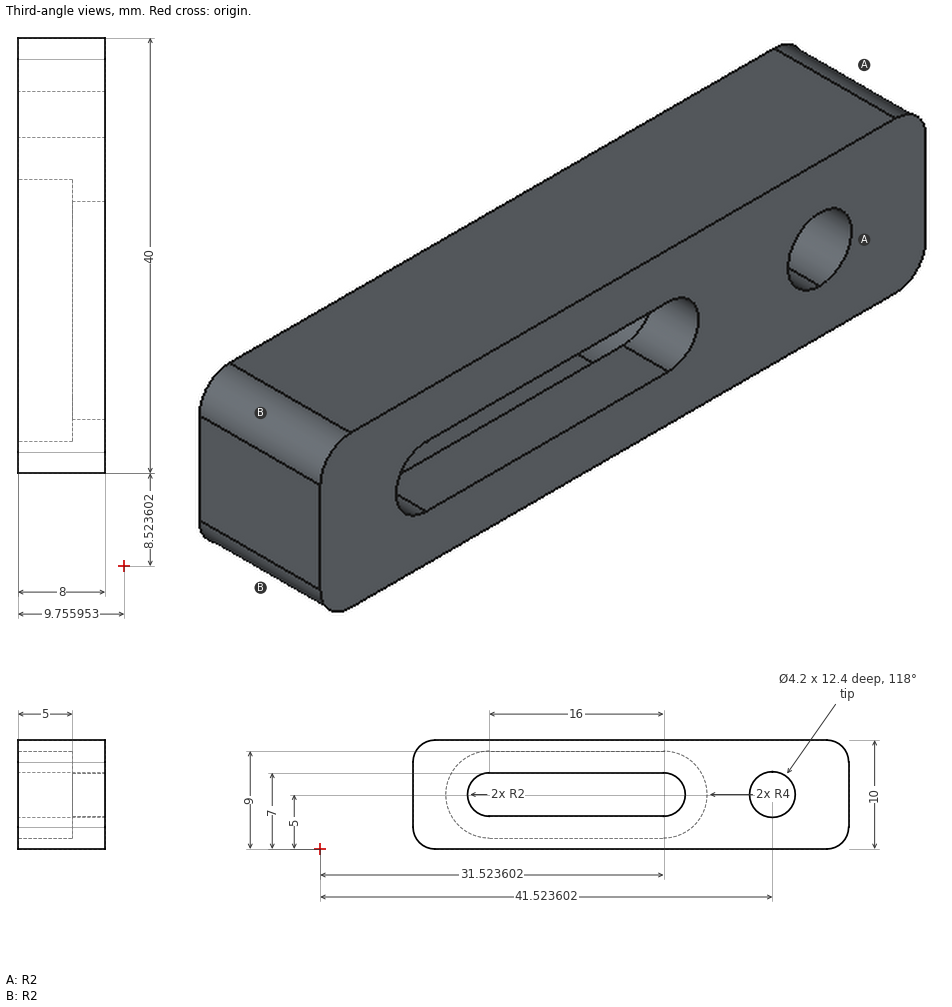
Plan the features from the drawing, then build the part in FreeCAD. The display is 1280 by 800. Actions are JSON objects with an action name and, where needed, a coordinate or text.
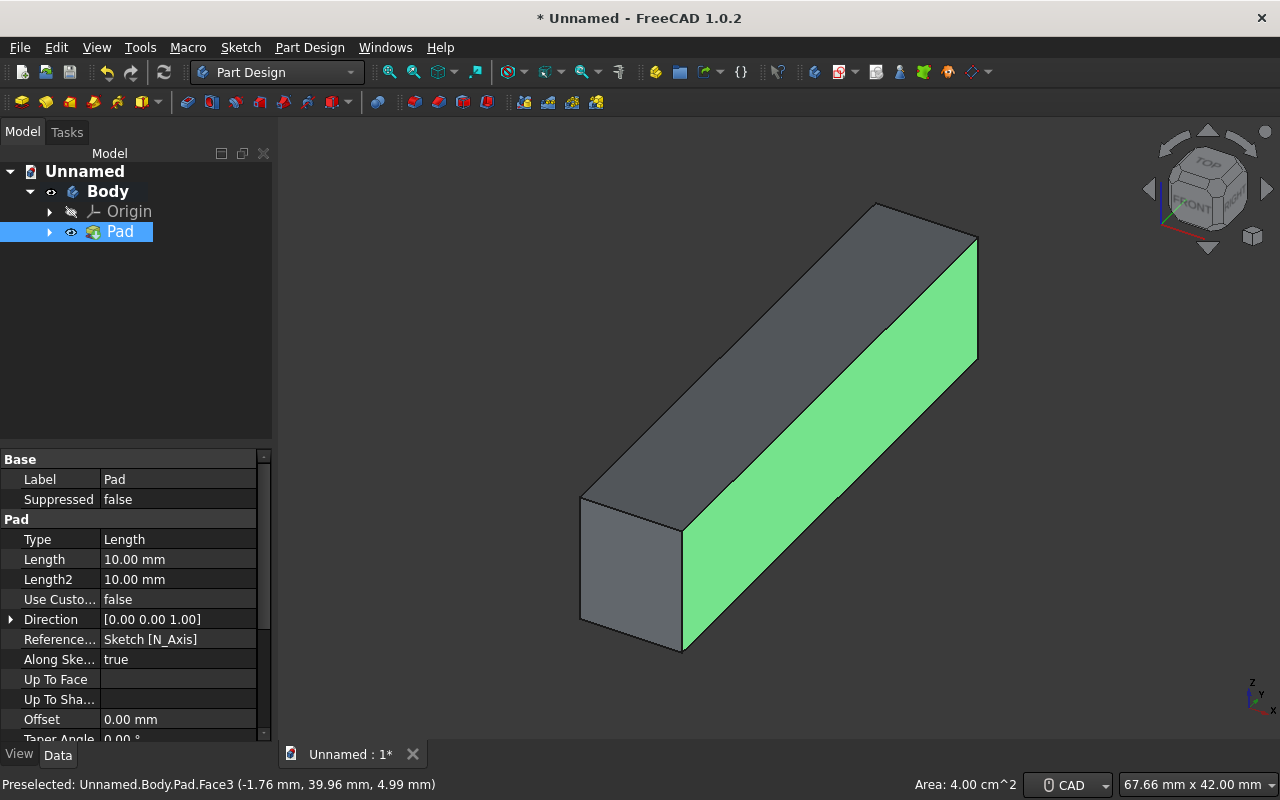
{"action": "left_click", "coordinate": [840, 72]}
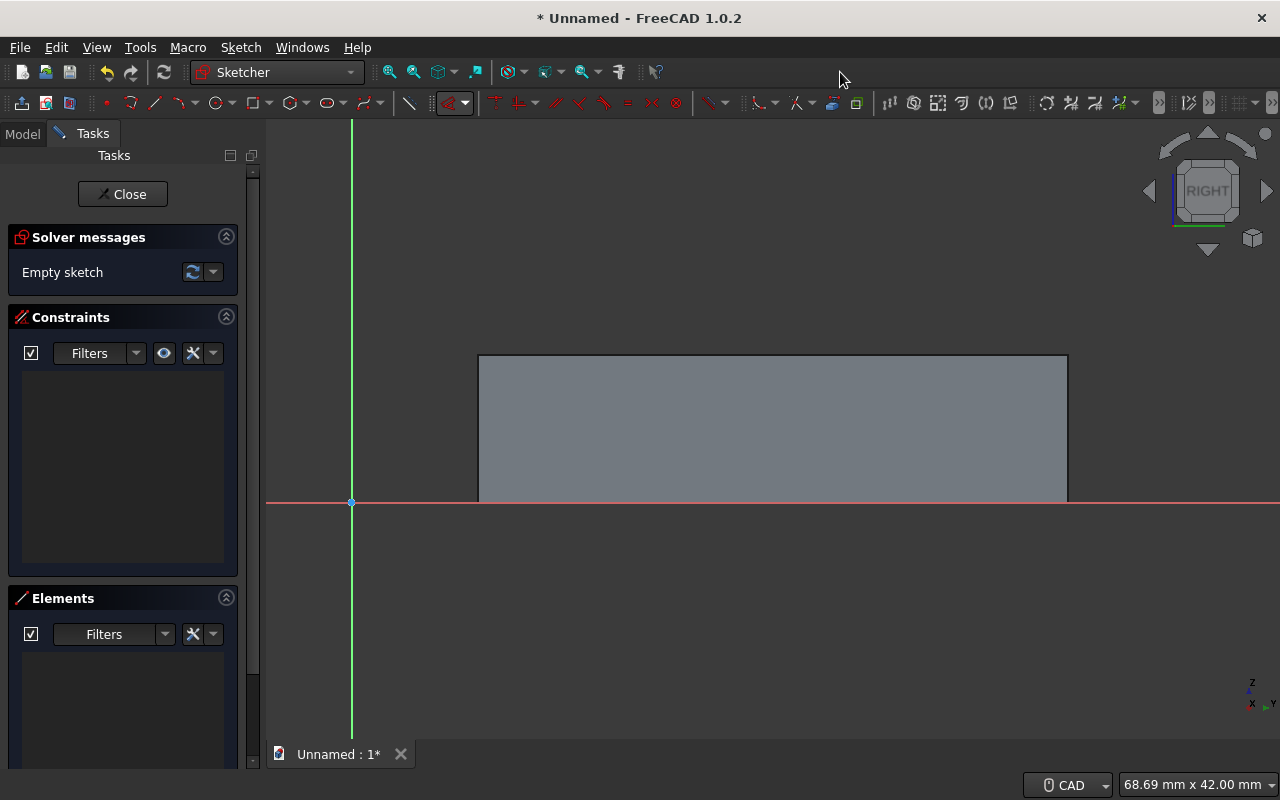
{"action": "scroll", "coordinate": [1016, 429], "scroll_direction": "up", "scroll_amount": 9}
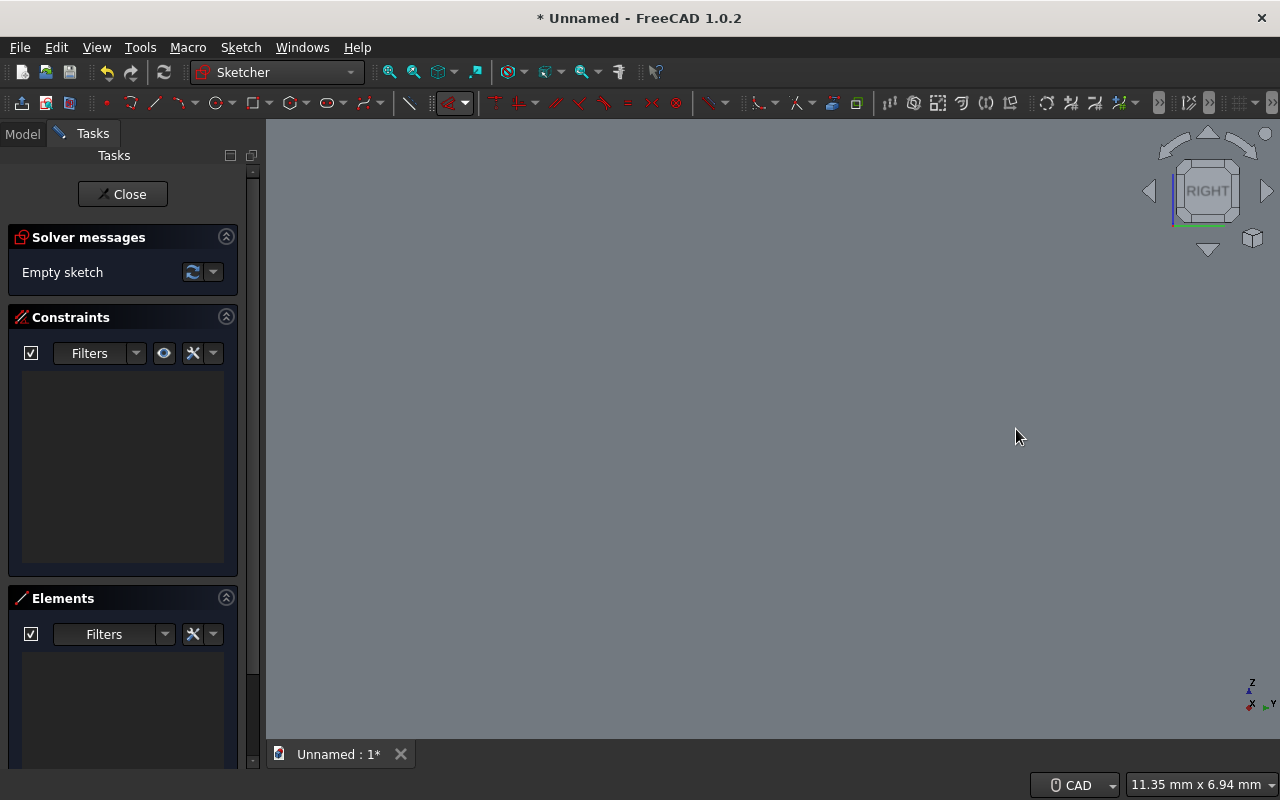
{"action": "left_click", "coordinate": [216, 104]}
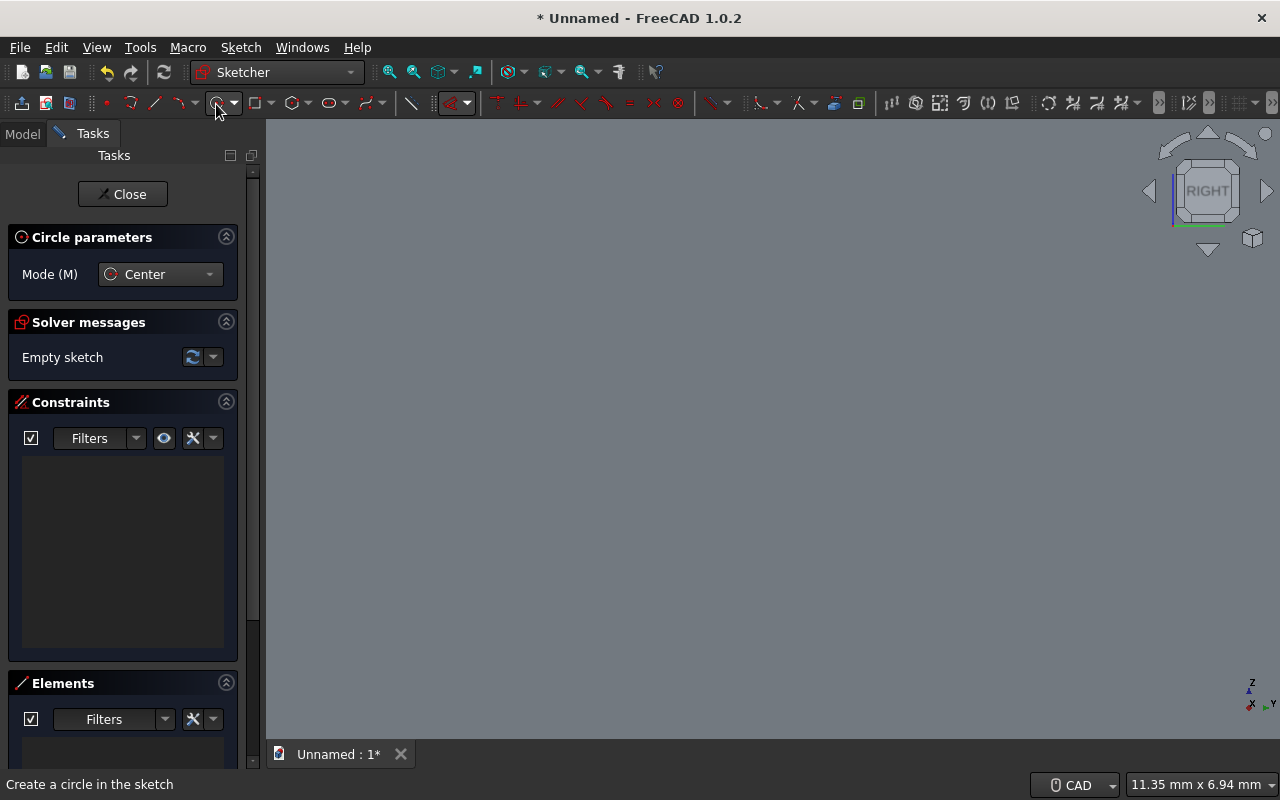
{"action": "left_click", "coordinate": [703, 426]}
{"action": "mouse_move", "coordinate": [836, 294]}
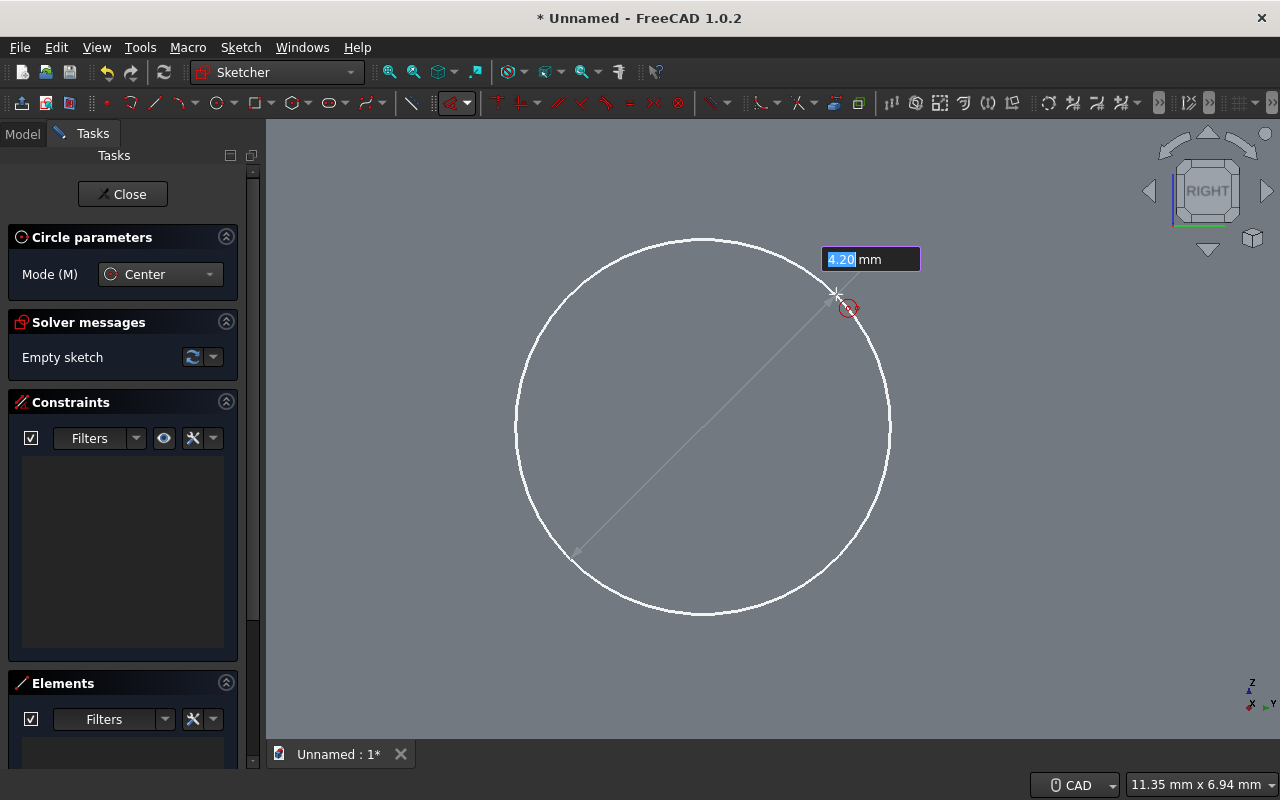
{"action": "type", "text": "4.2"}
{"action": "key", "text": "Return"}
{"action": "key", "text": "Escape"}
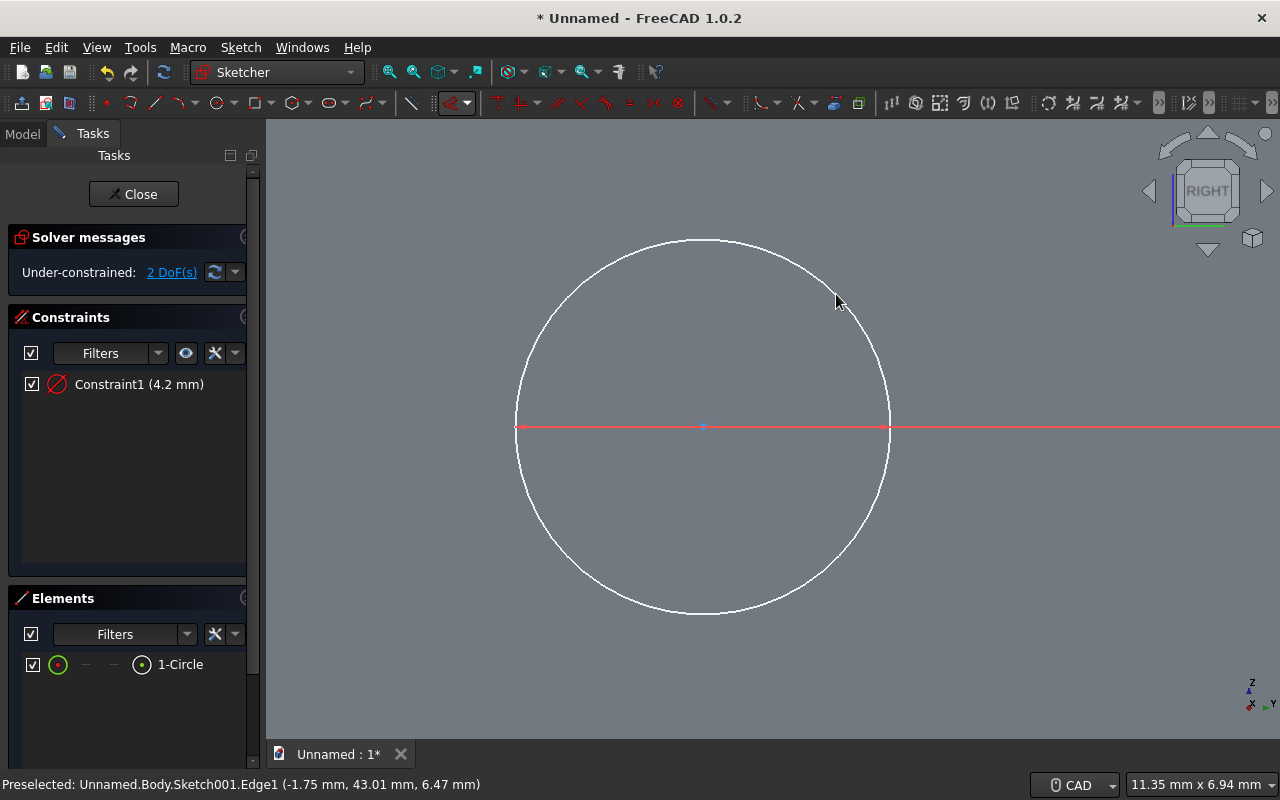
{"action": "key", "text": "d"}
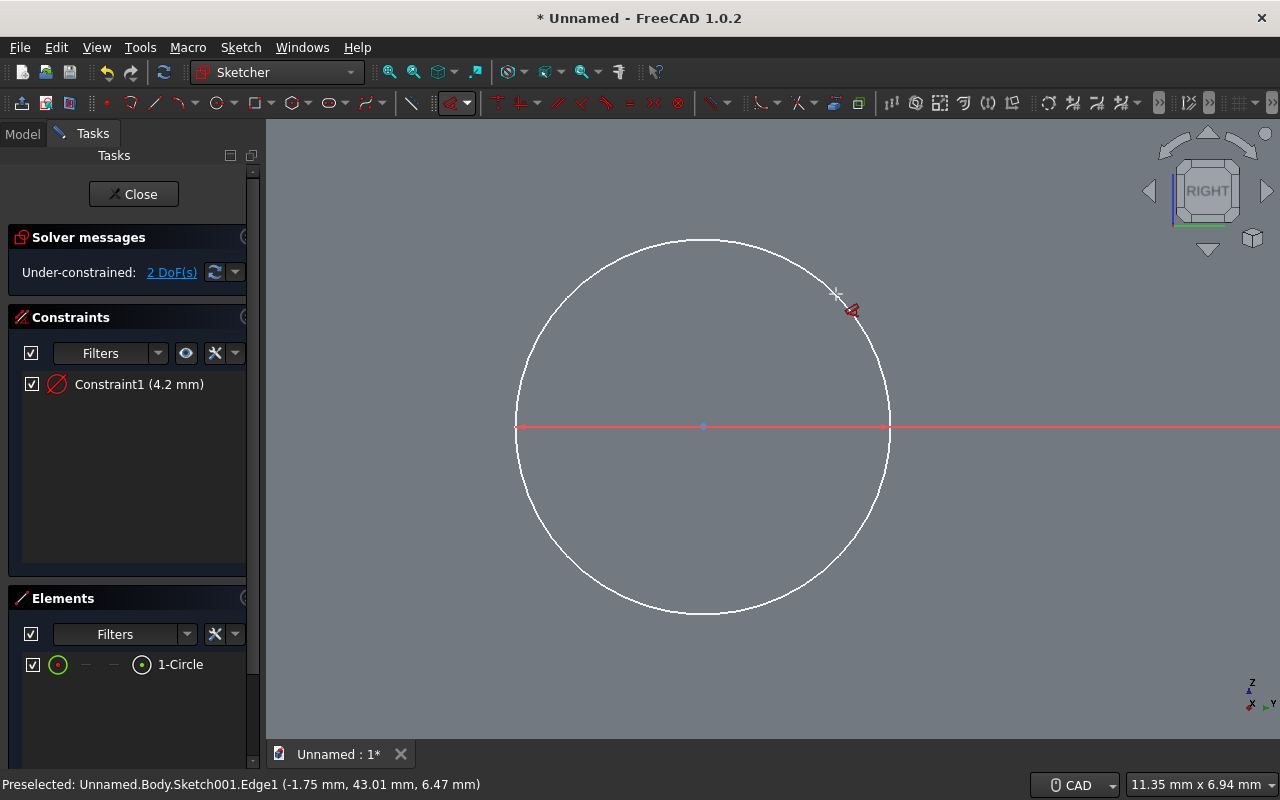
{"action": "left_click", "coordinate": [703, 427]}
{"action": "left_click", "coordinate": [737, 569]}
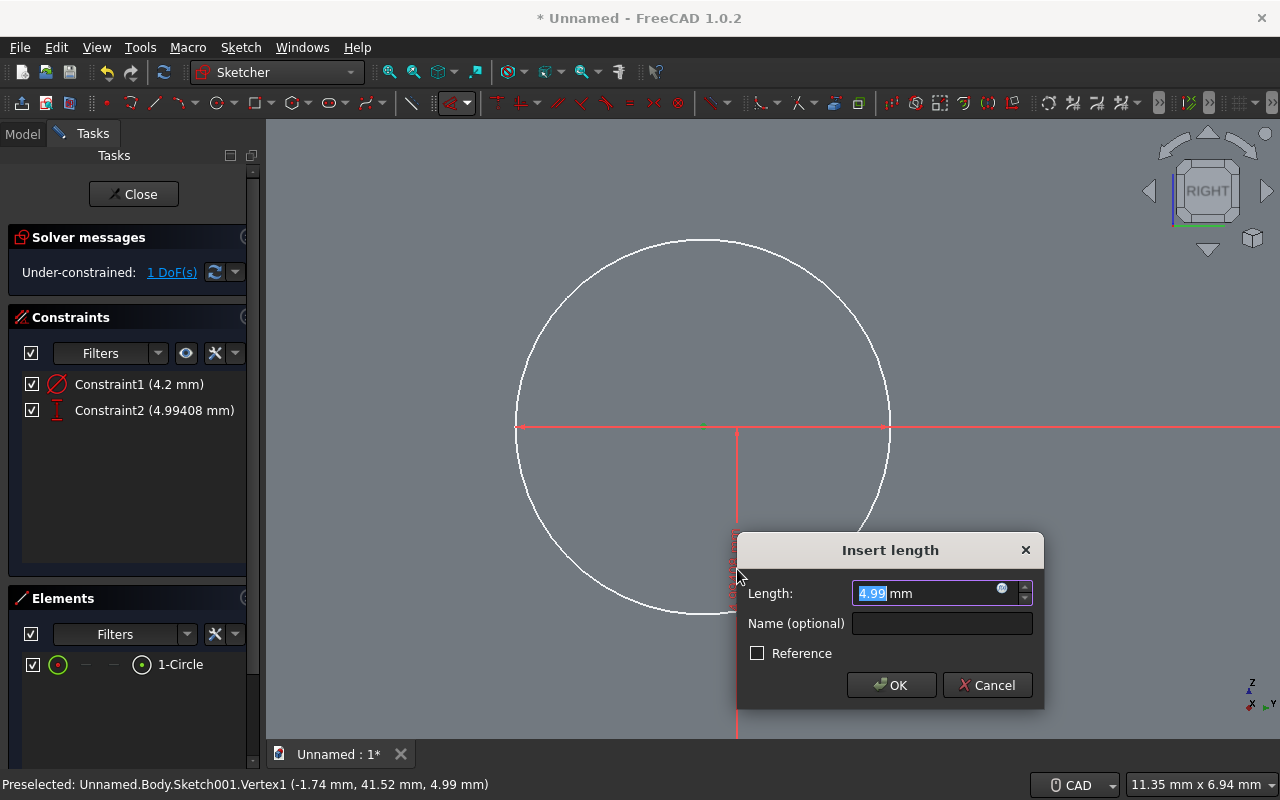
{"action": "type", "text": "5"}
{"action": "key", "text": "Return"}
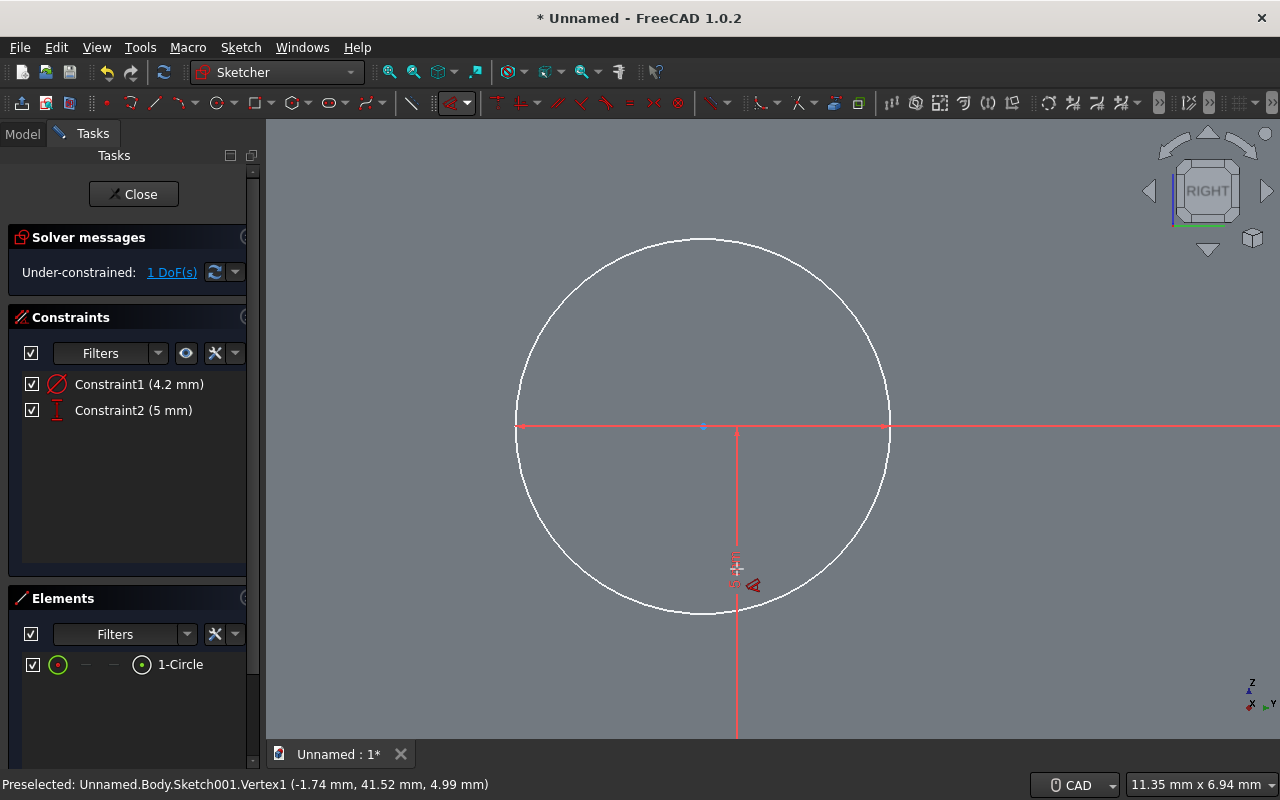
{"action": "left_click", "coordinate": [703, 426]}
{"action": "left_click", "coordinate": [499, 392]}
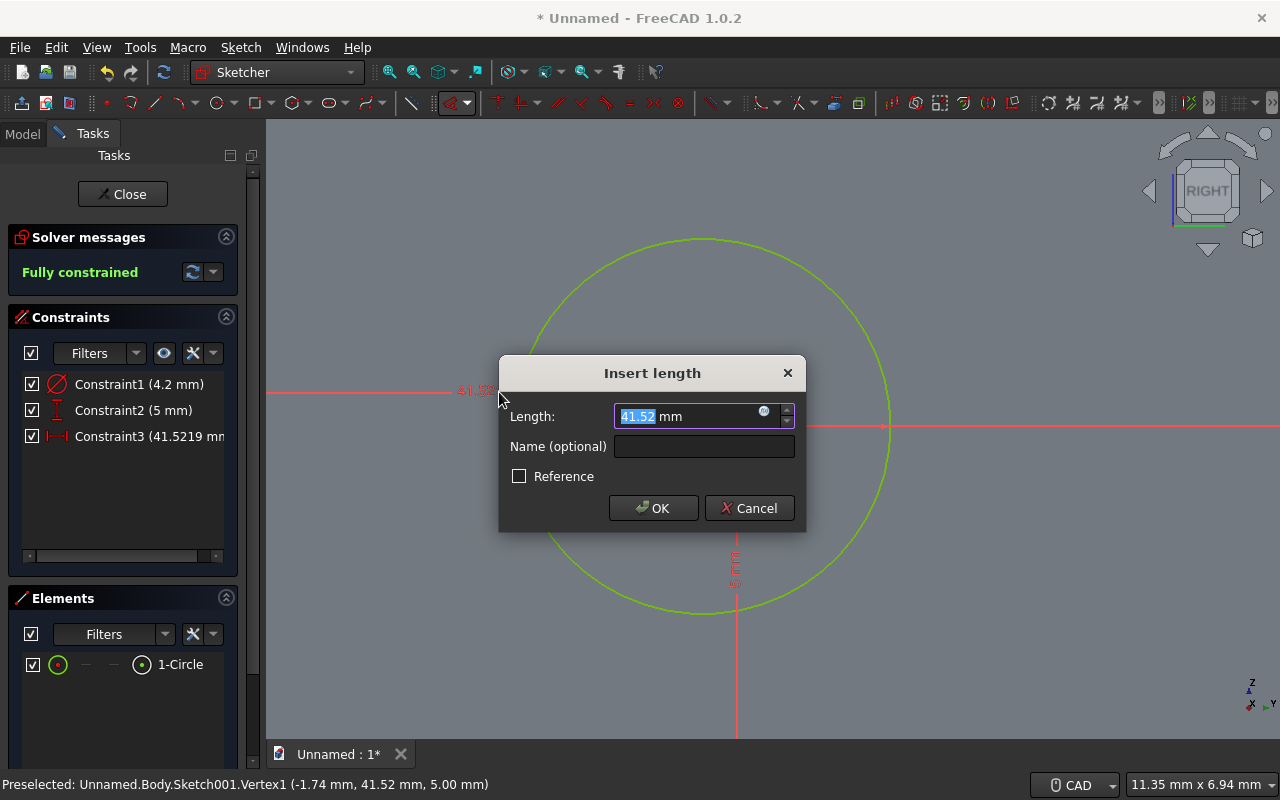
{"action": "type", "text": "41.523602"}
{"action": "key", "text": "Return"}
{"action": "key", "text": "Escape"}